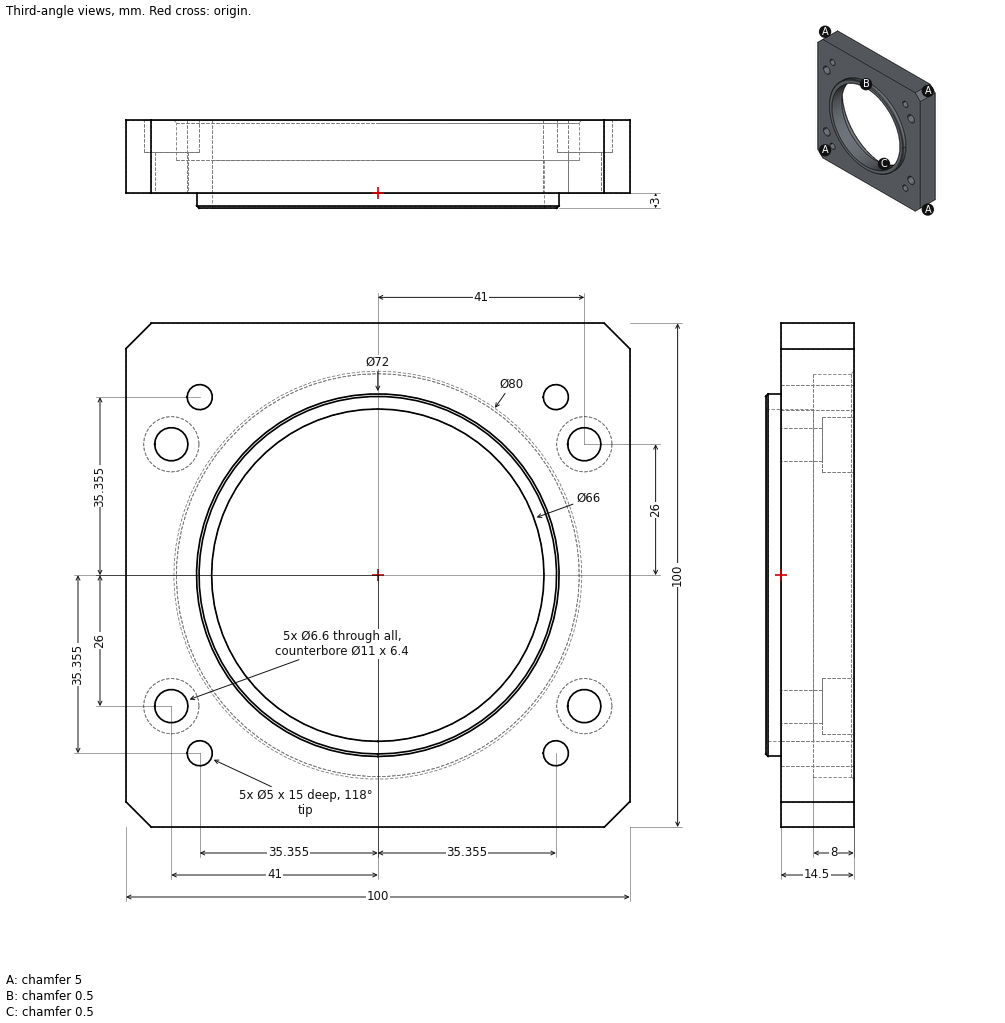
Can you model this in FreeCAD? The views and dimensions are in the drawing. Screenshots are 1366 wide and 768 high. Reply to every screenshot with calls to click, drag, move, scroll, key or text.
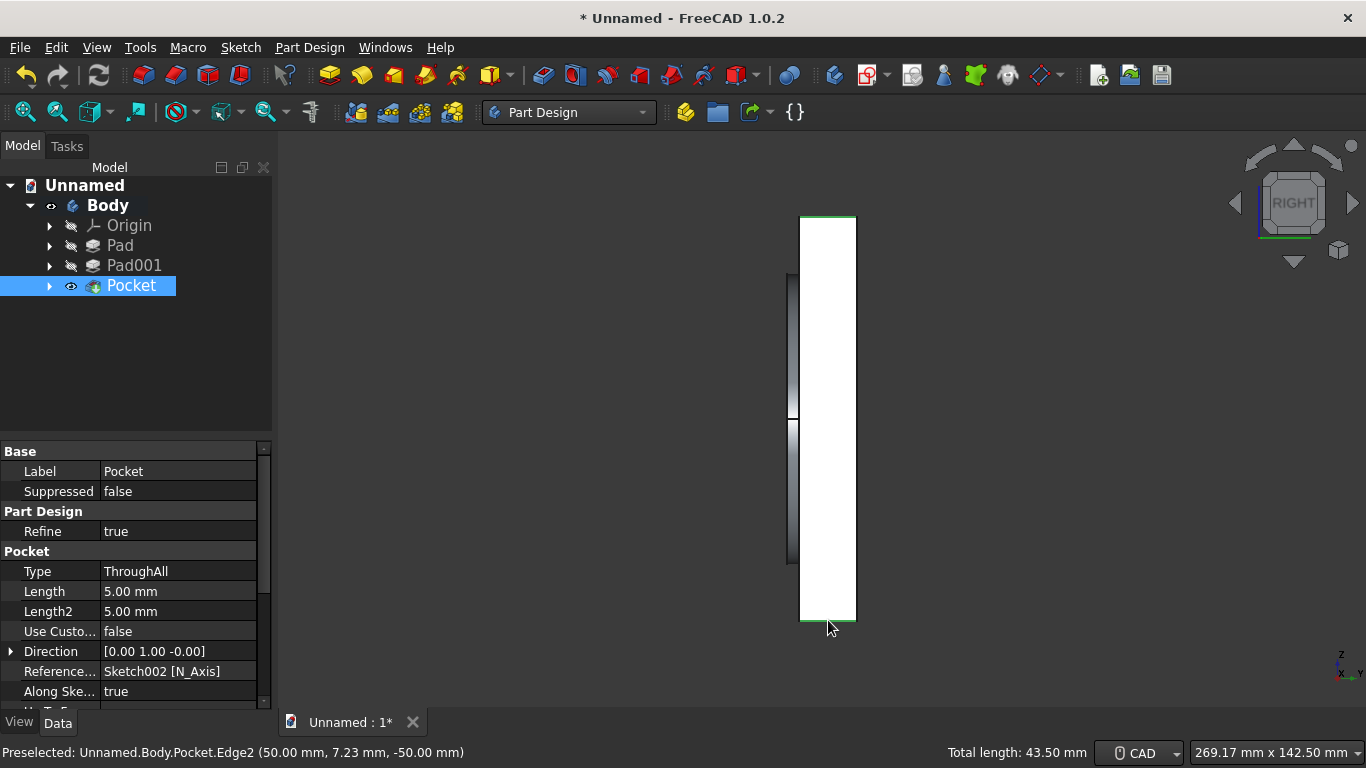
key(5)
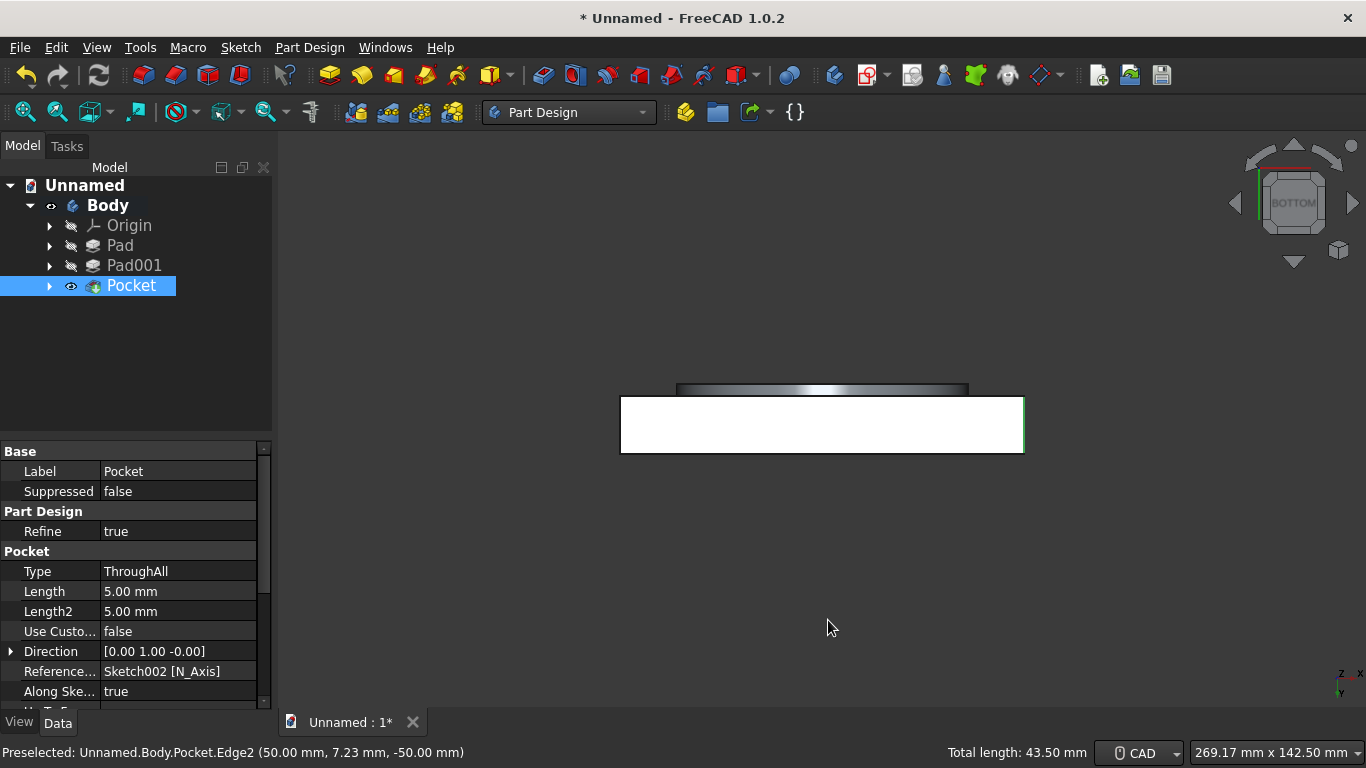
key(v)
key(f)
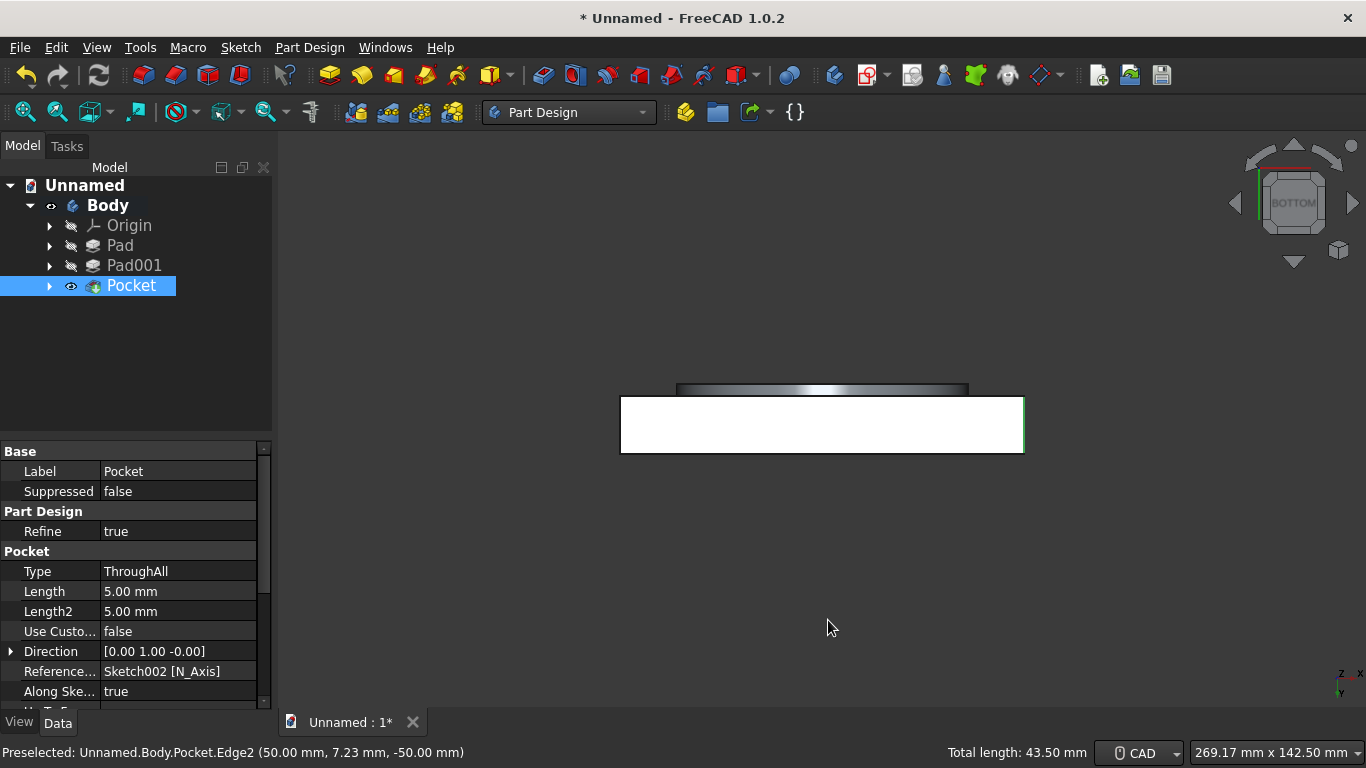
click(620, 424, ctrl)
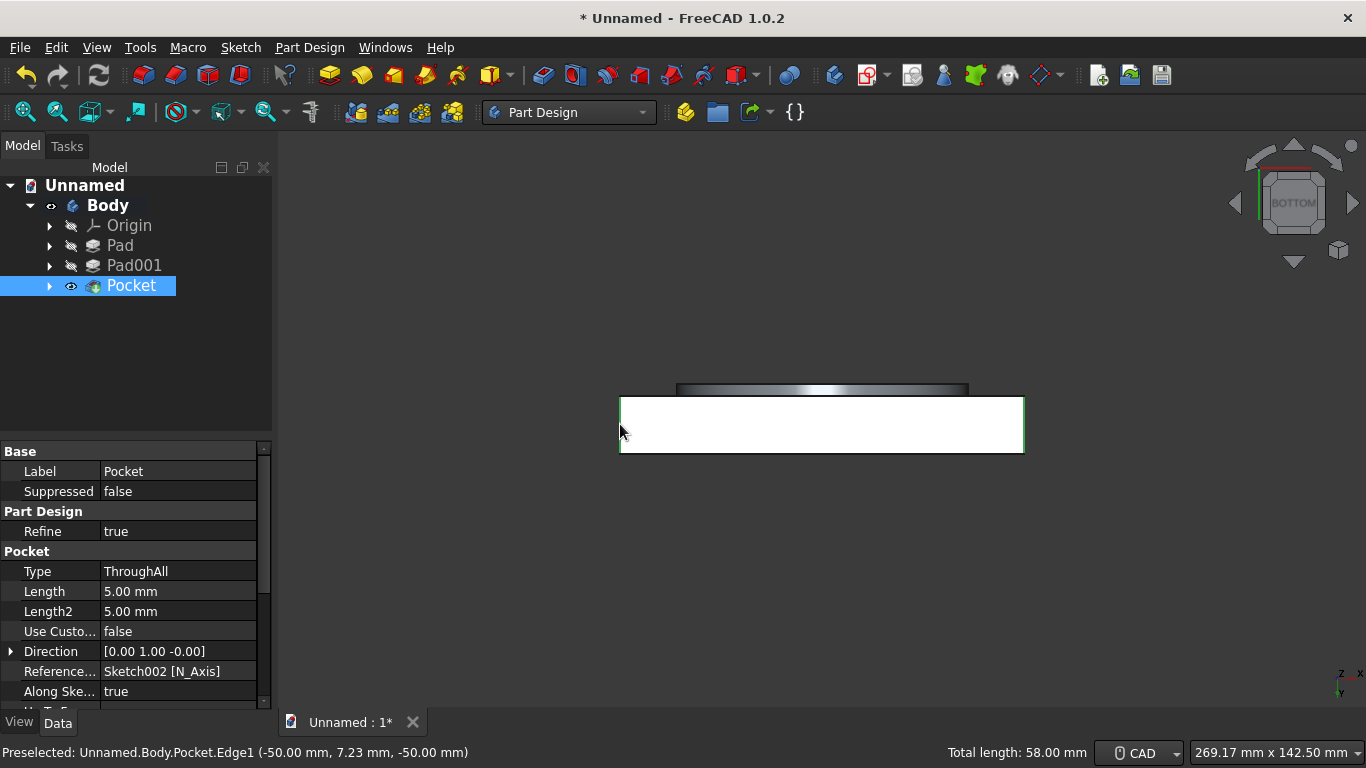
click(176, 76)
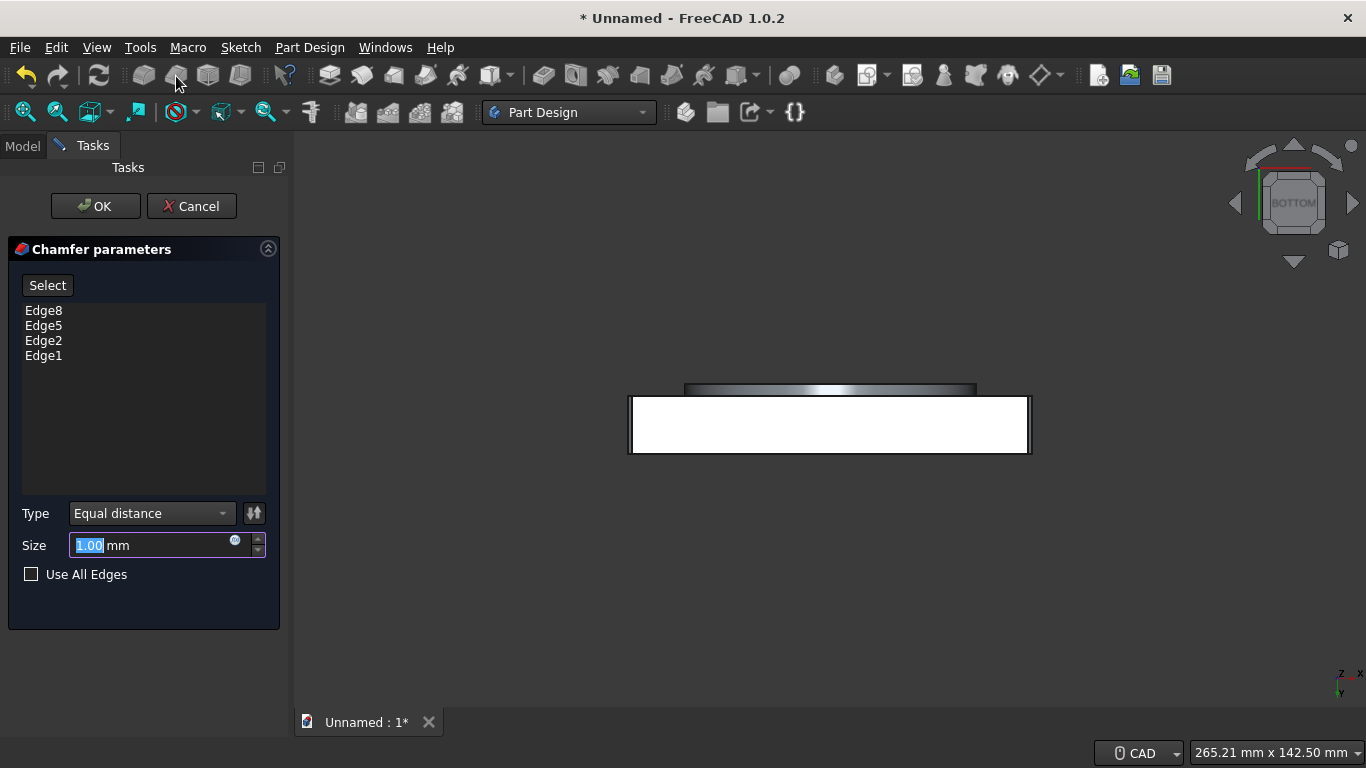
text(5)
key(Tab)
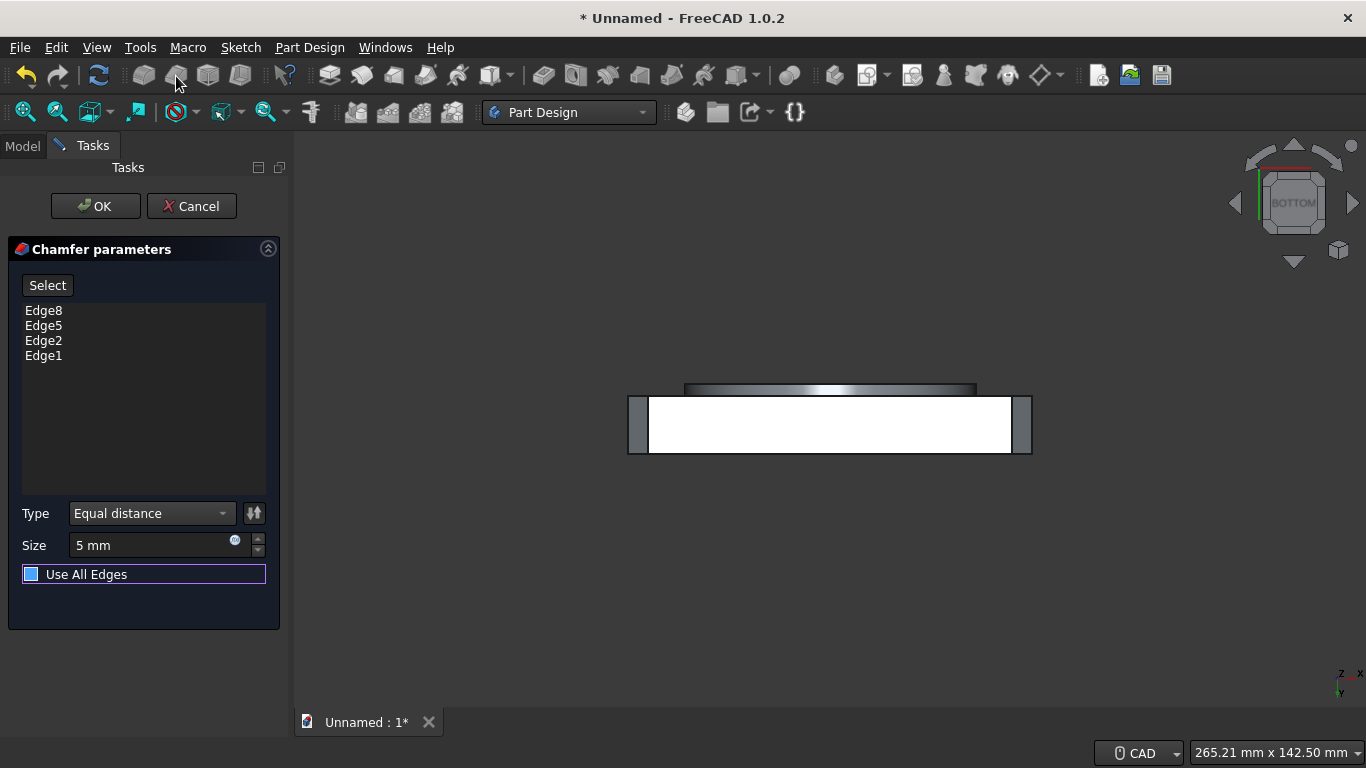
click(96, 206)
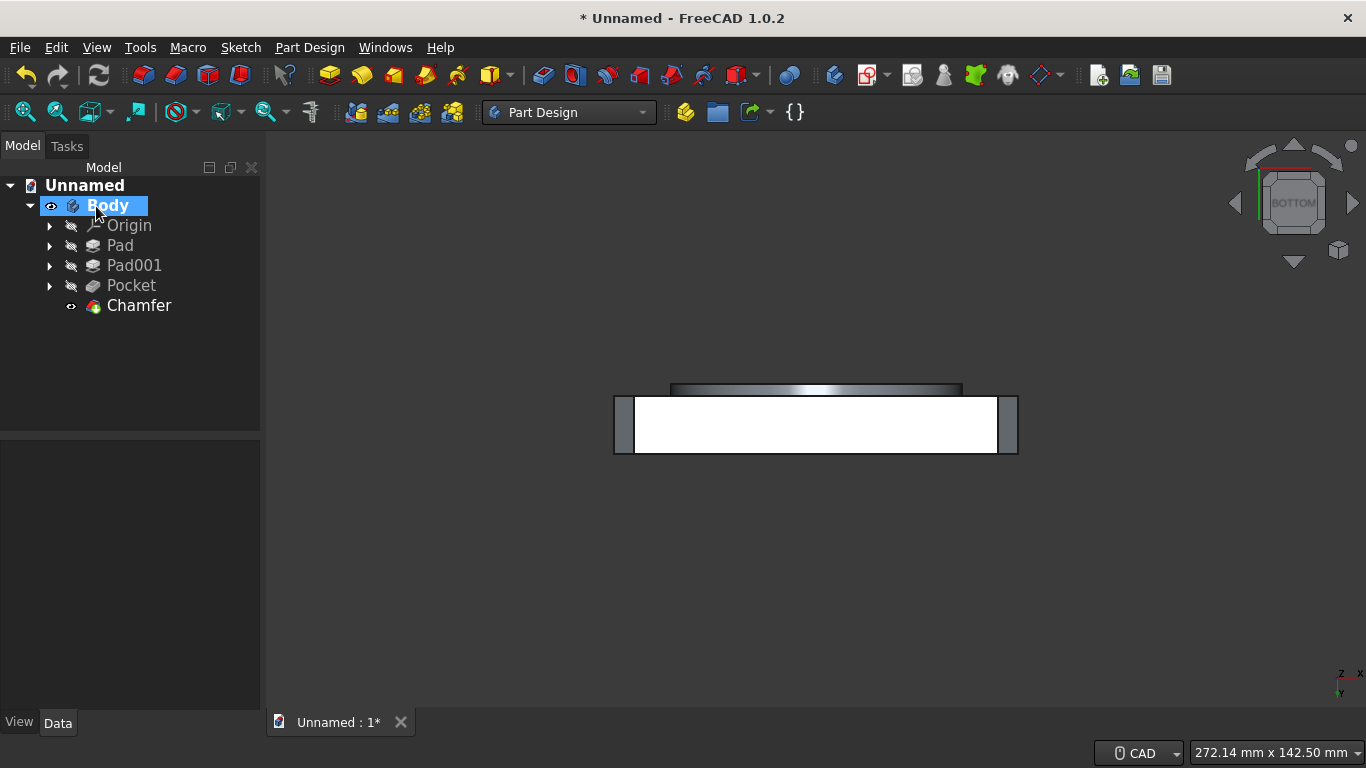
click(26, 112)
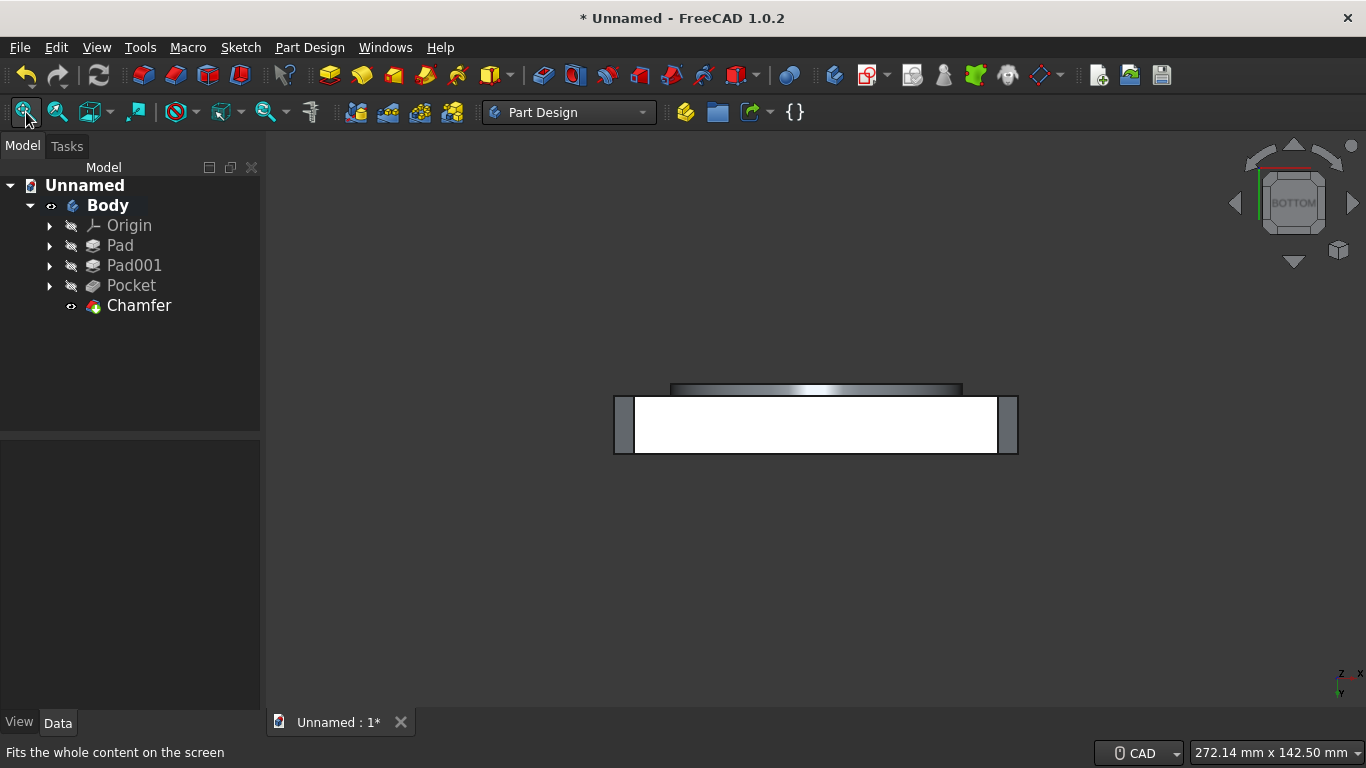
click(698, 383)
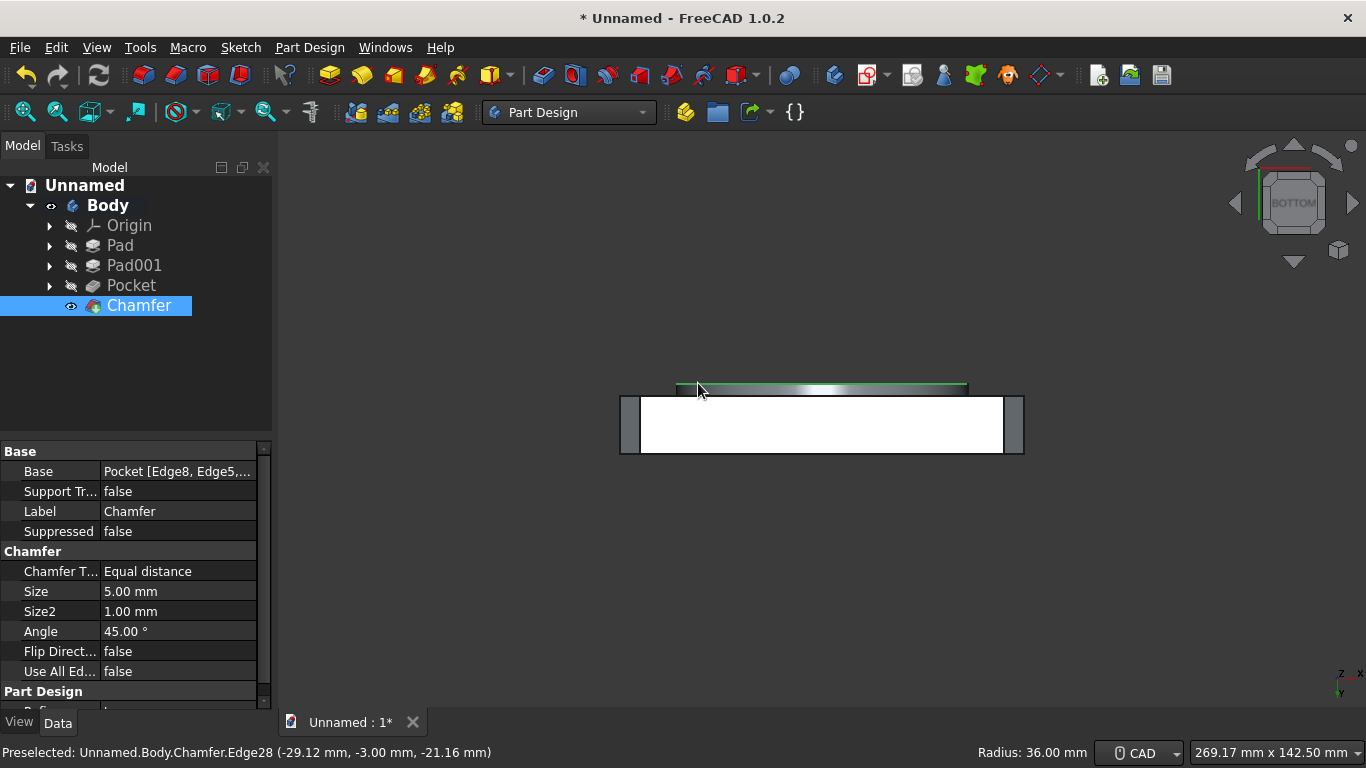
click(176, 76)